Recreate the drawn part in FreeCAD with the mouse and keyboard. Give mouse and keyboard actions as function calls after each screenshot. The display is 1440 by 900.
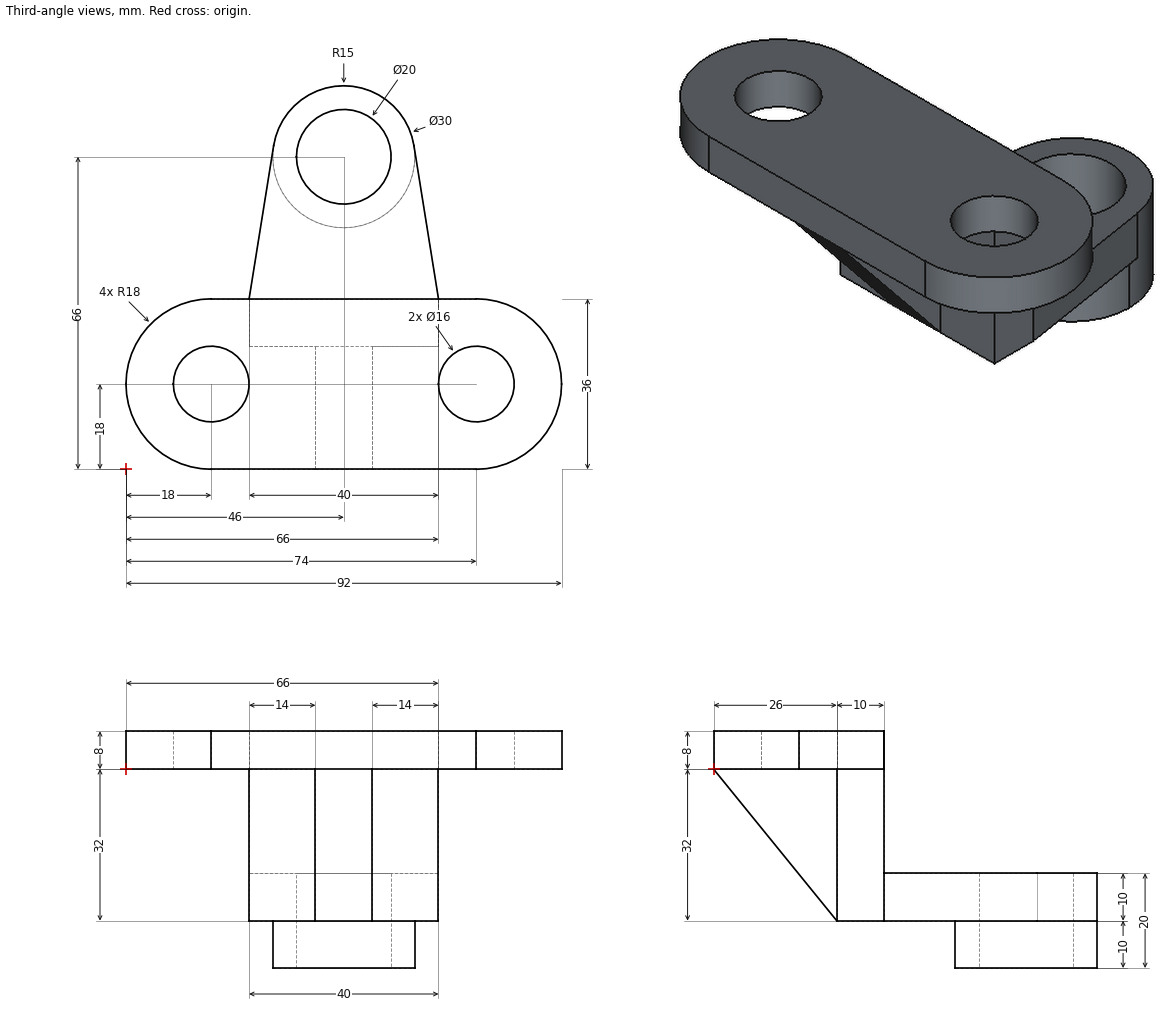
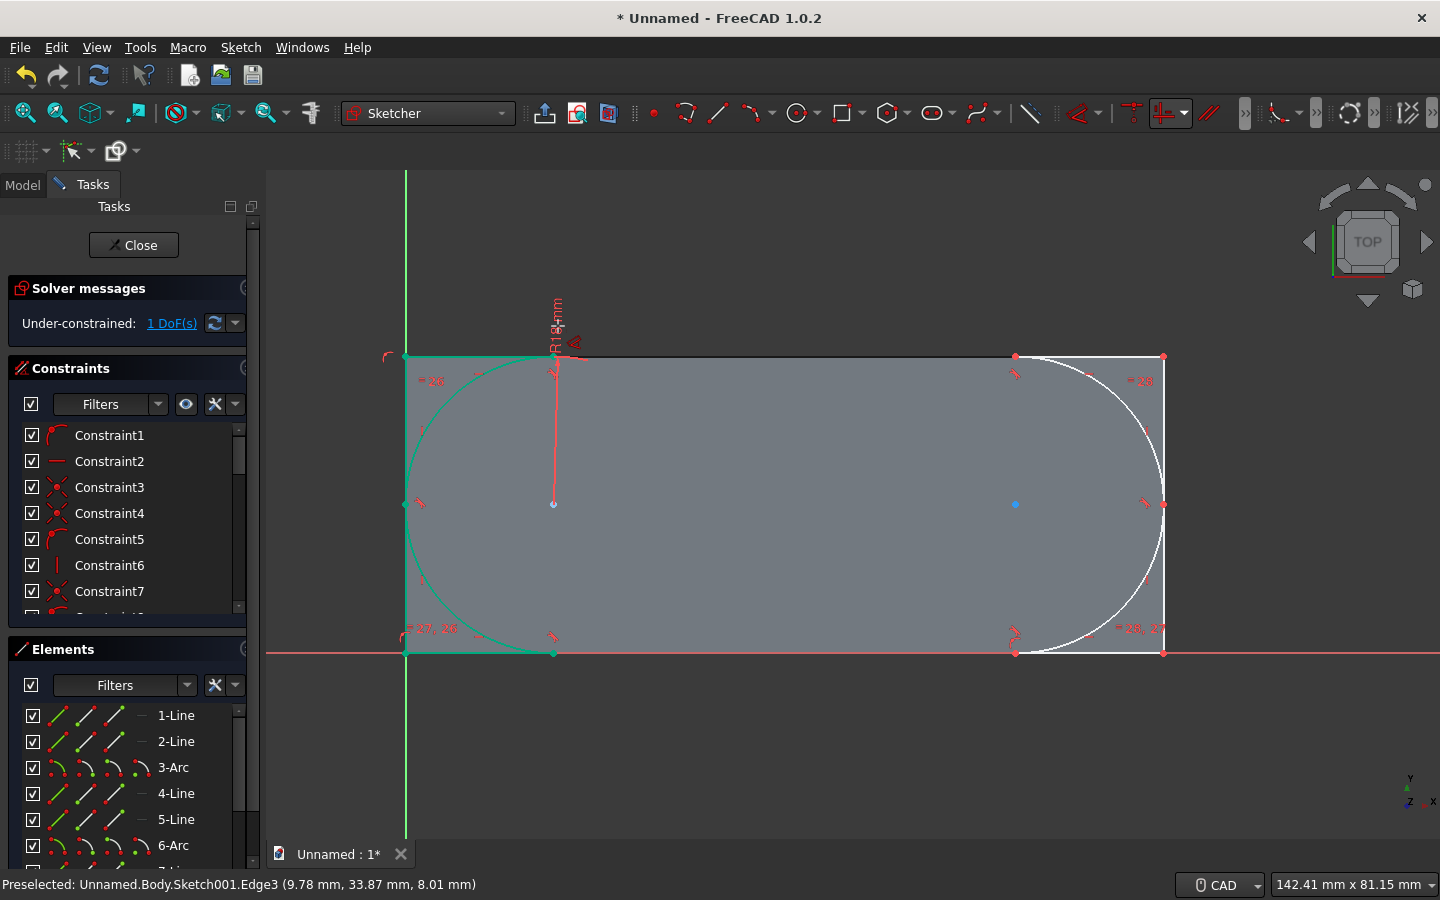
click(1016, 653)
click(711, 687)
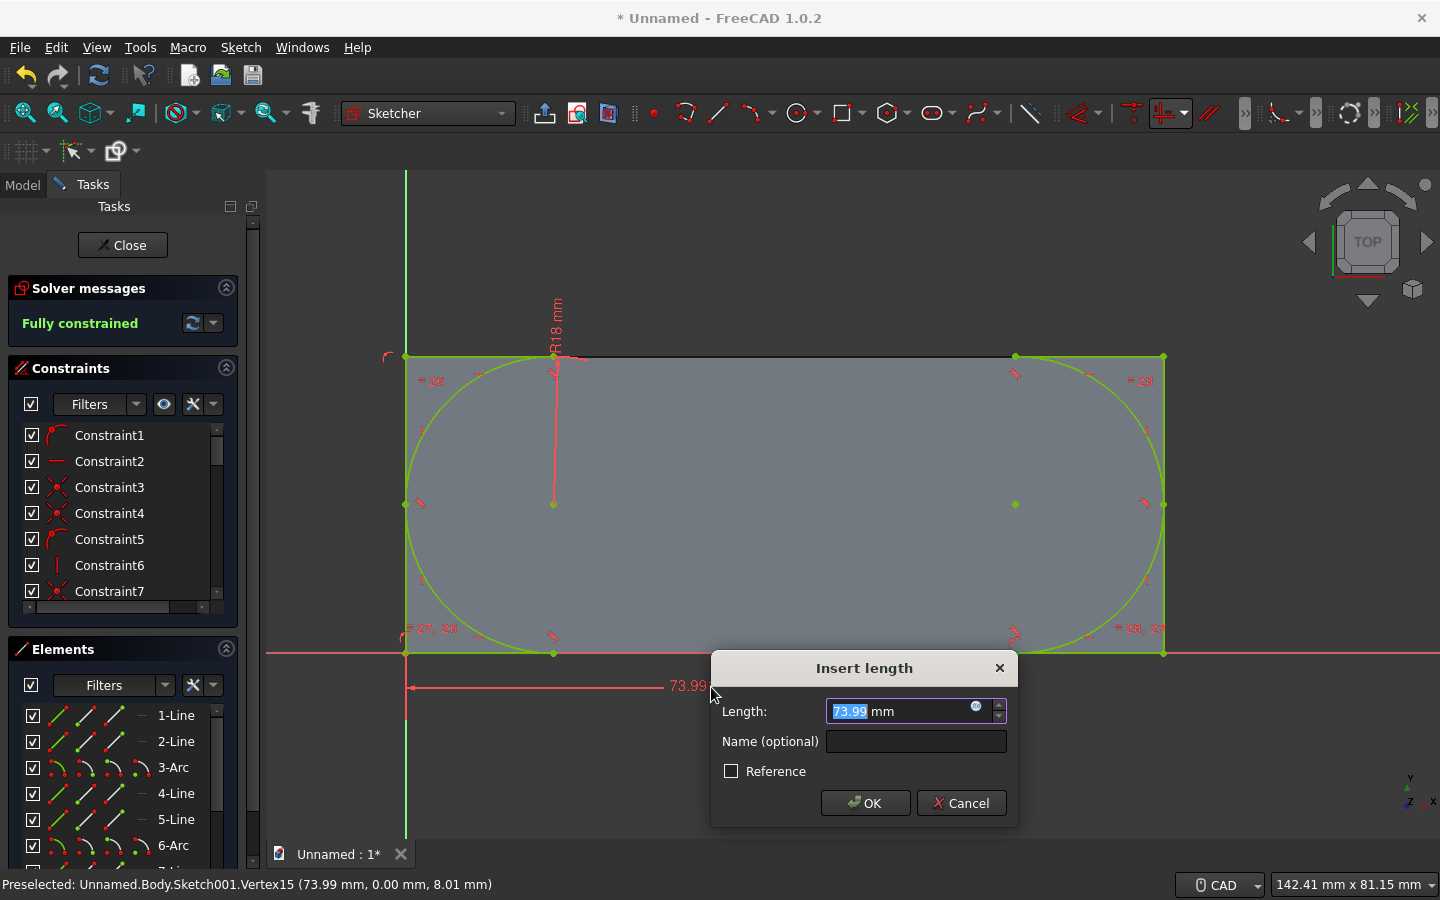
text(74)
key(Return)
key(Escape)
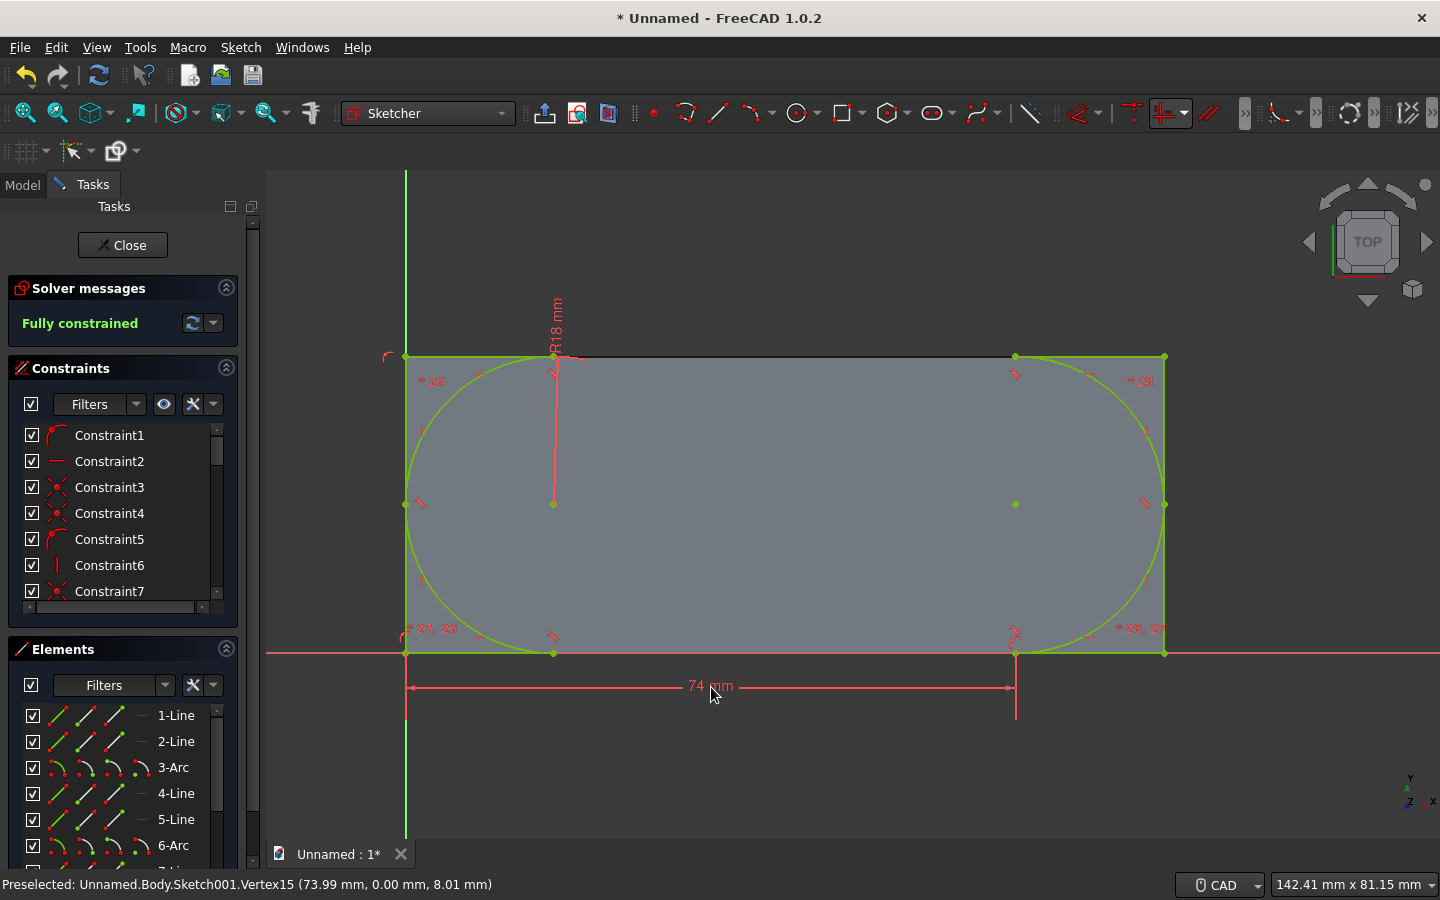
click(123, 245)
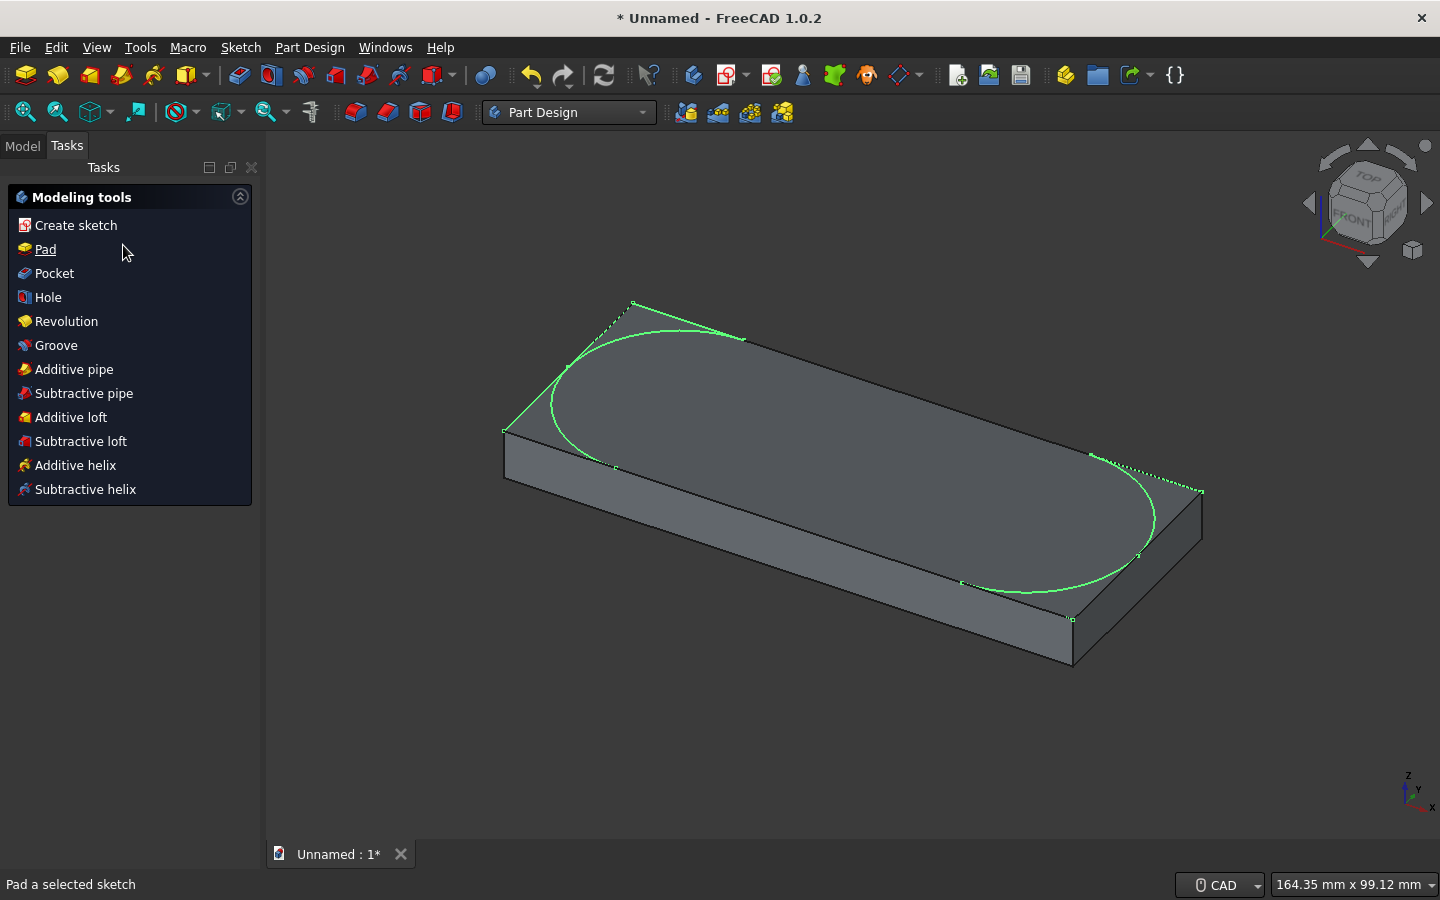
click(240, 76)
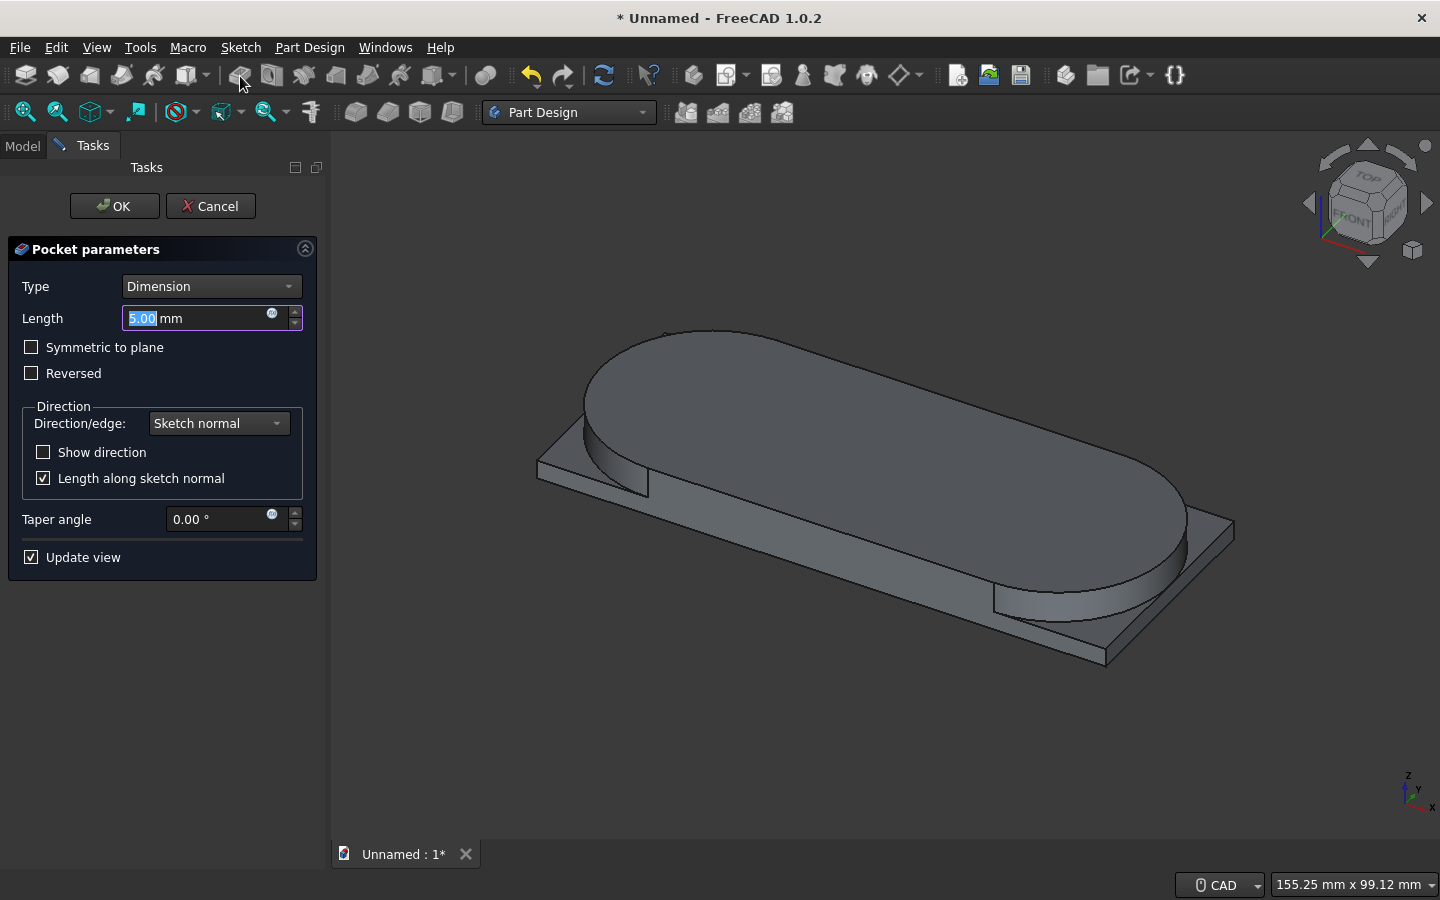
text(8)
key(Tab)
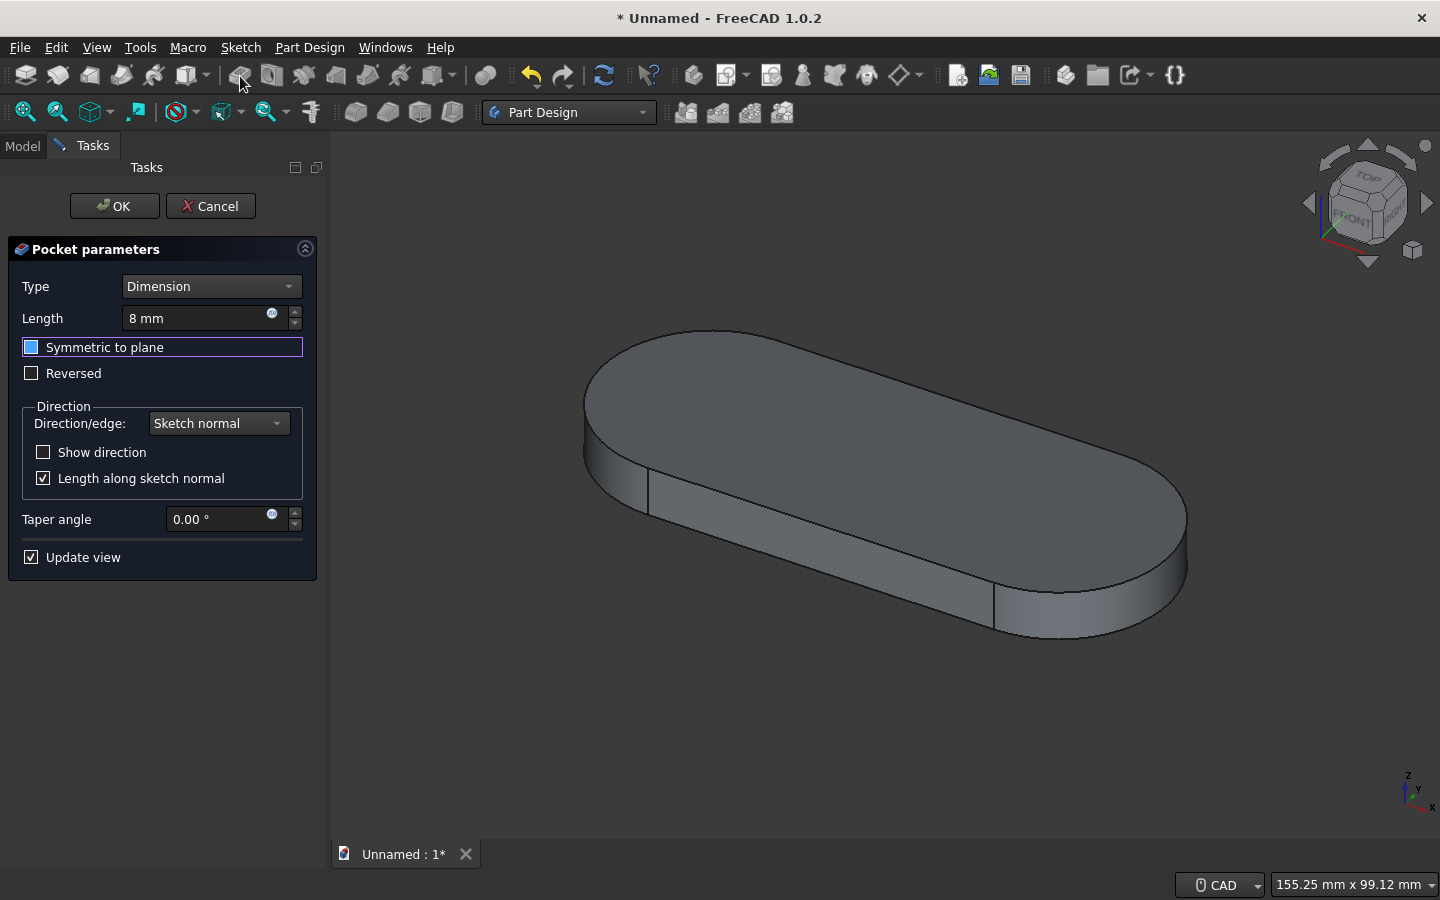
click(115, 206)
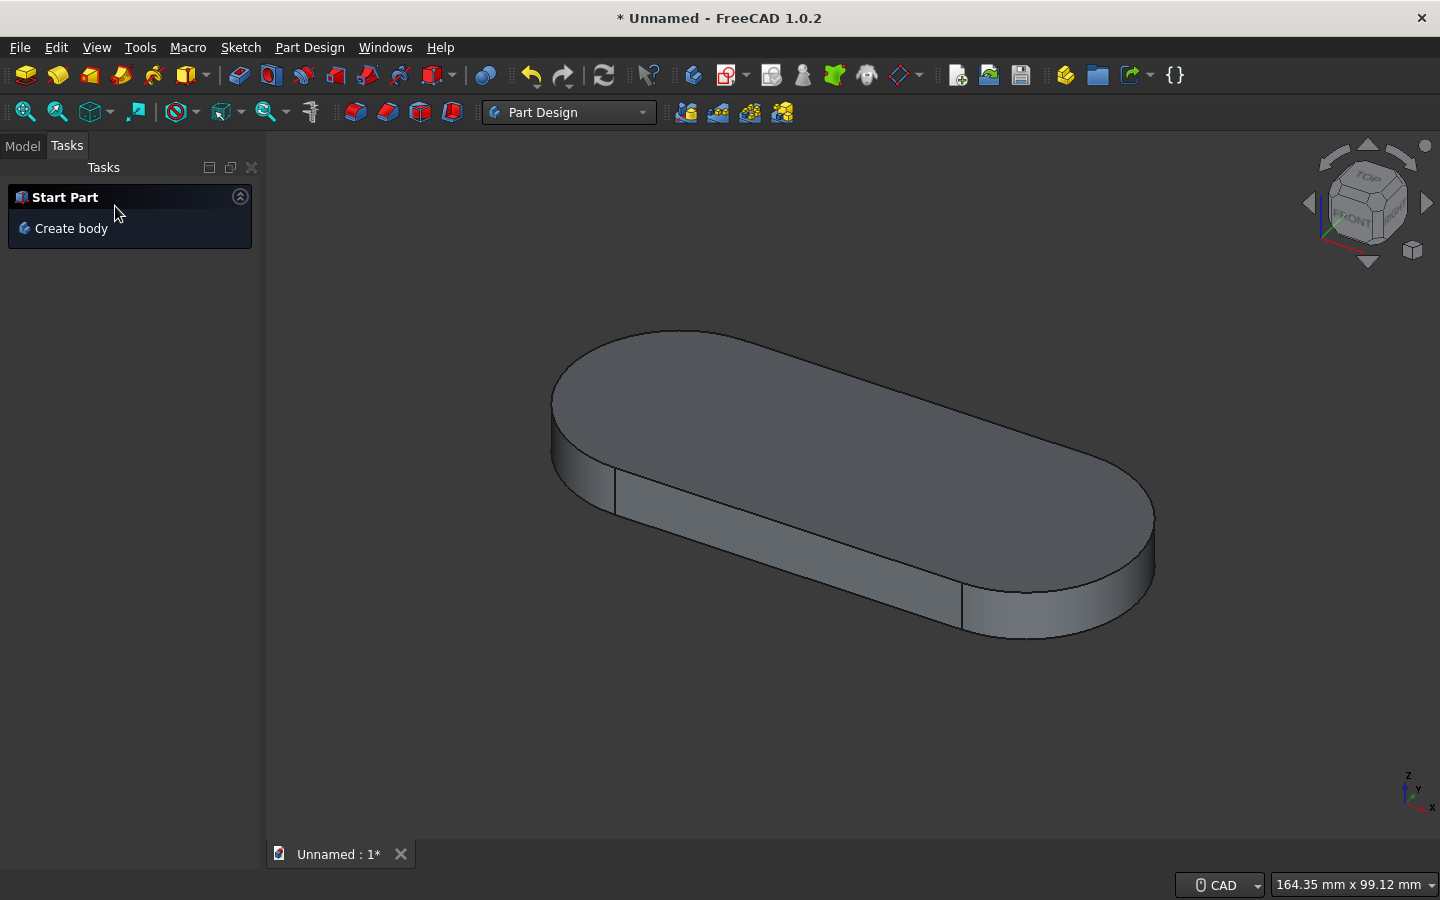
key(4)